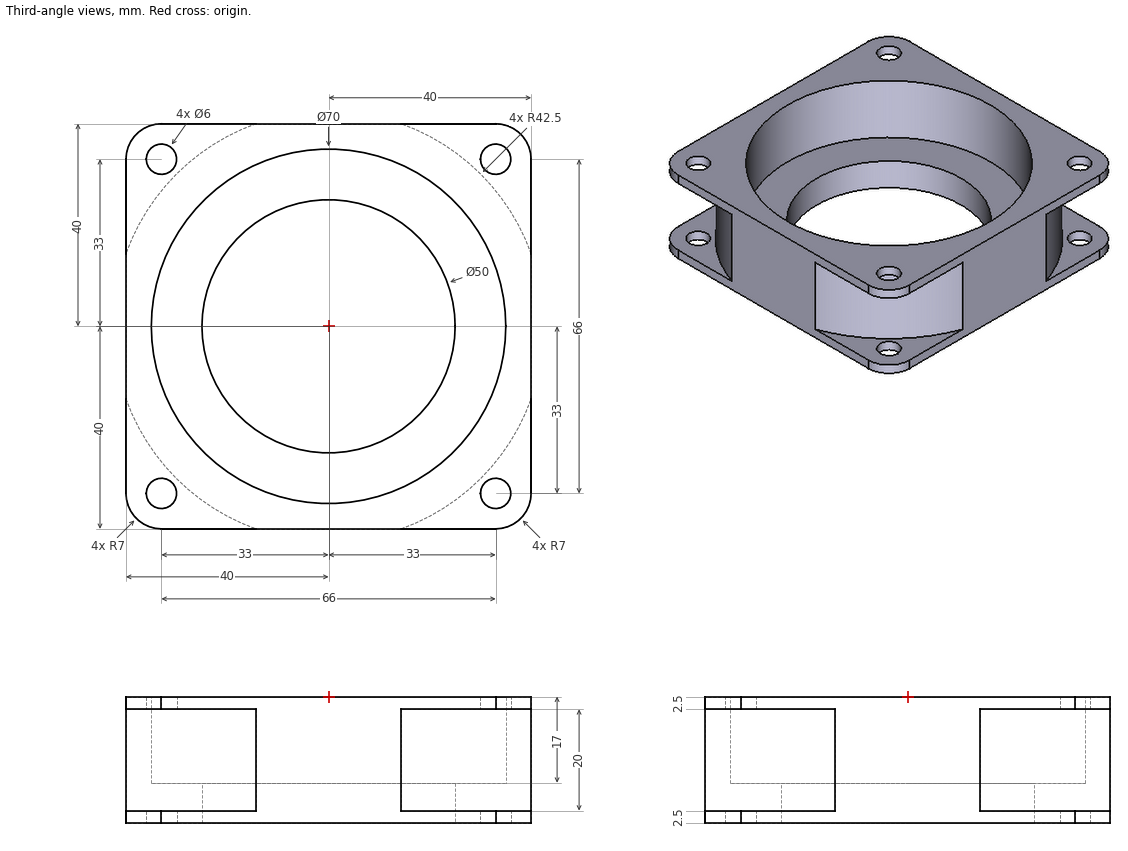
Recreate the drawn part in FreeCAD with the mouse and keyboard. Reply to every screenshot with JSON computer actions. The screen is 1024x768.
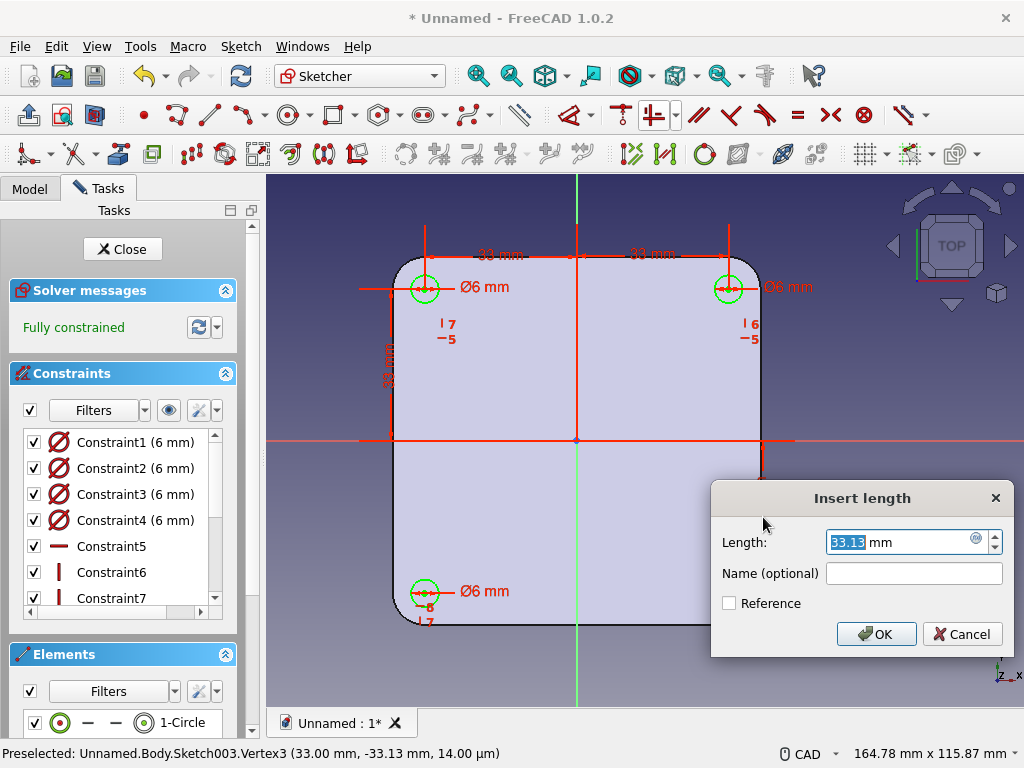
{"action": "type", "text": "33"}
{"action": "key", "text": "Return"}
{"action": "key", "text": "Escape"}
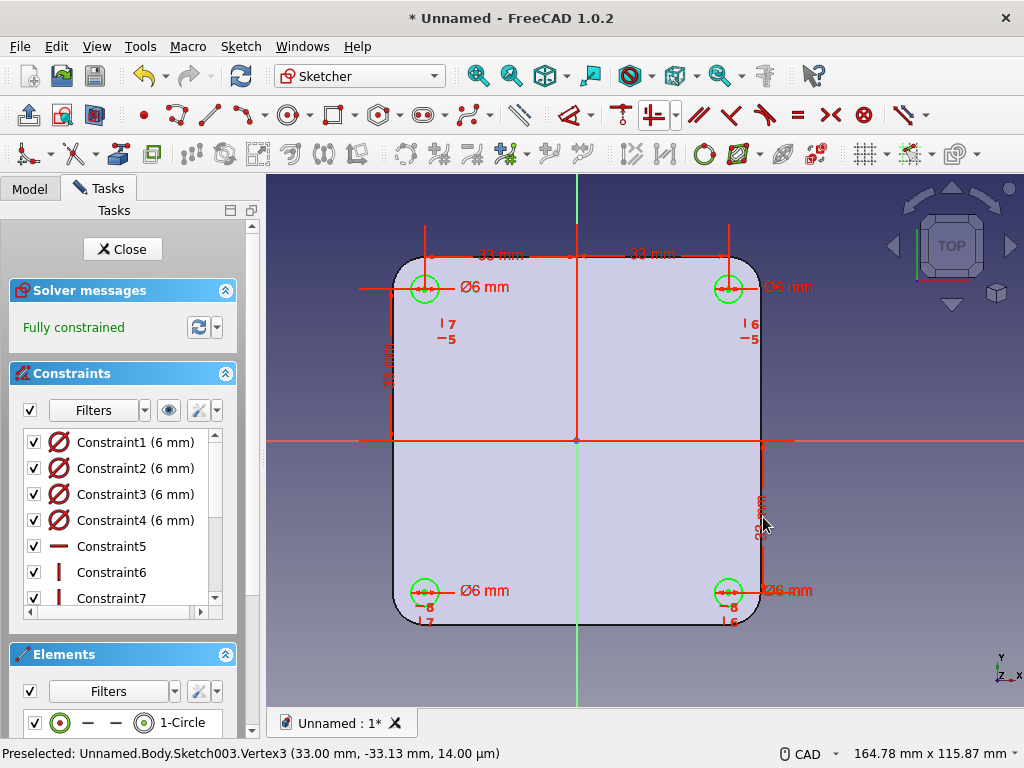
{"action": "left_click", "coordinate": [123, 249]}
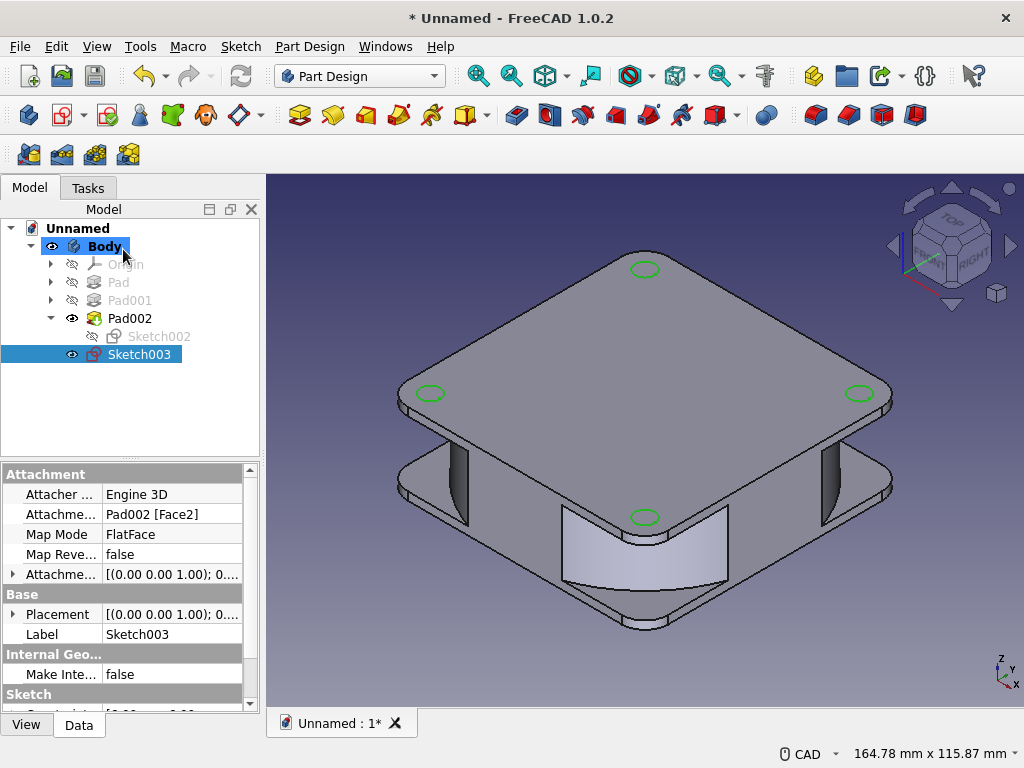
{"action": "left_click", "coordinate": [517, 116]}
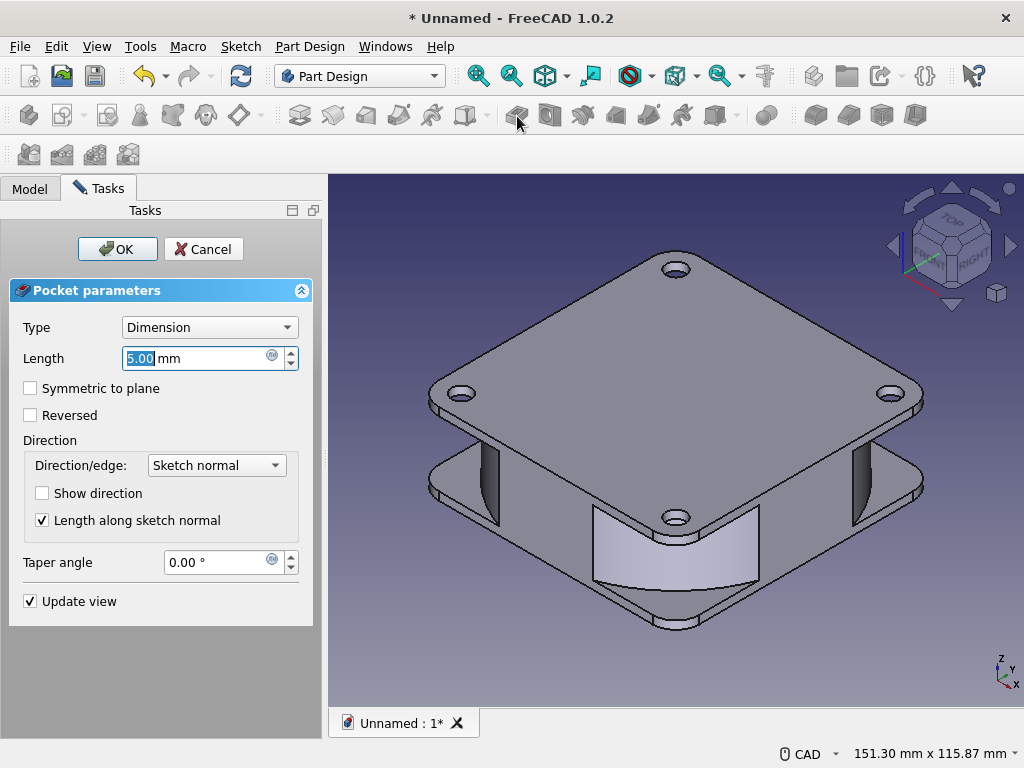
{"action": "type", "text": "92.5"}
{"action": "key", "text": "Tab"}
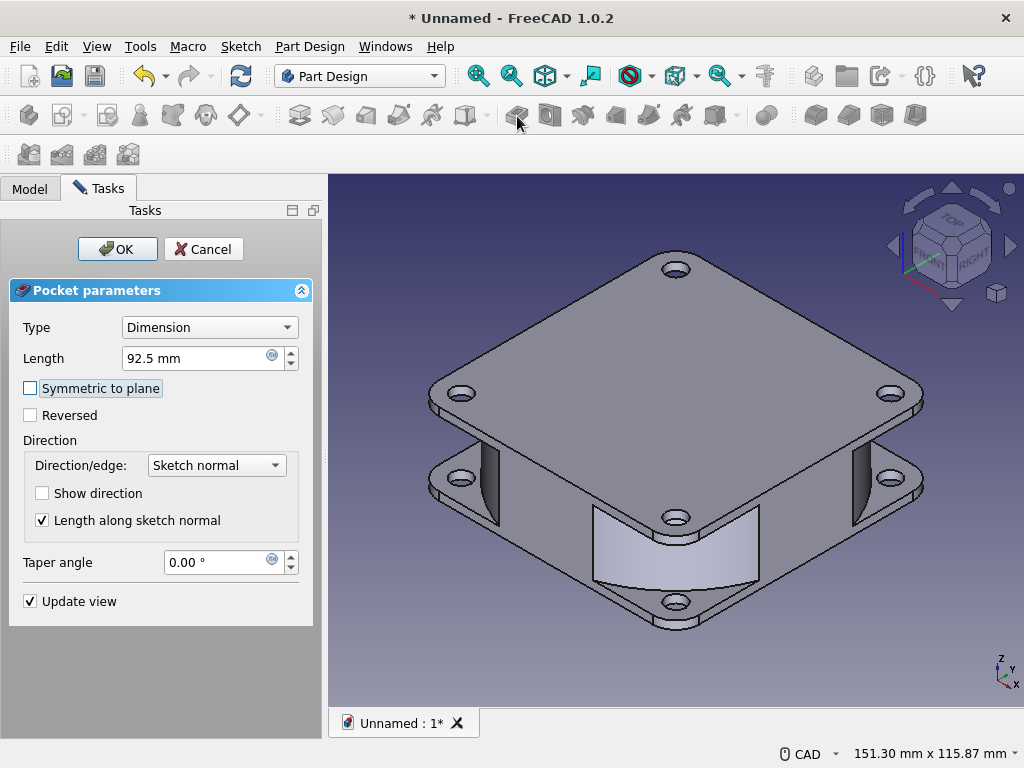
{"action": "left_click", "coordinate": [118, 249]}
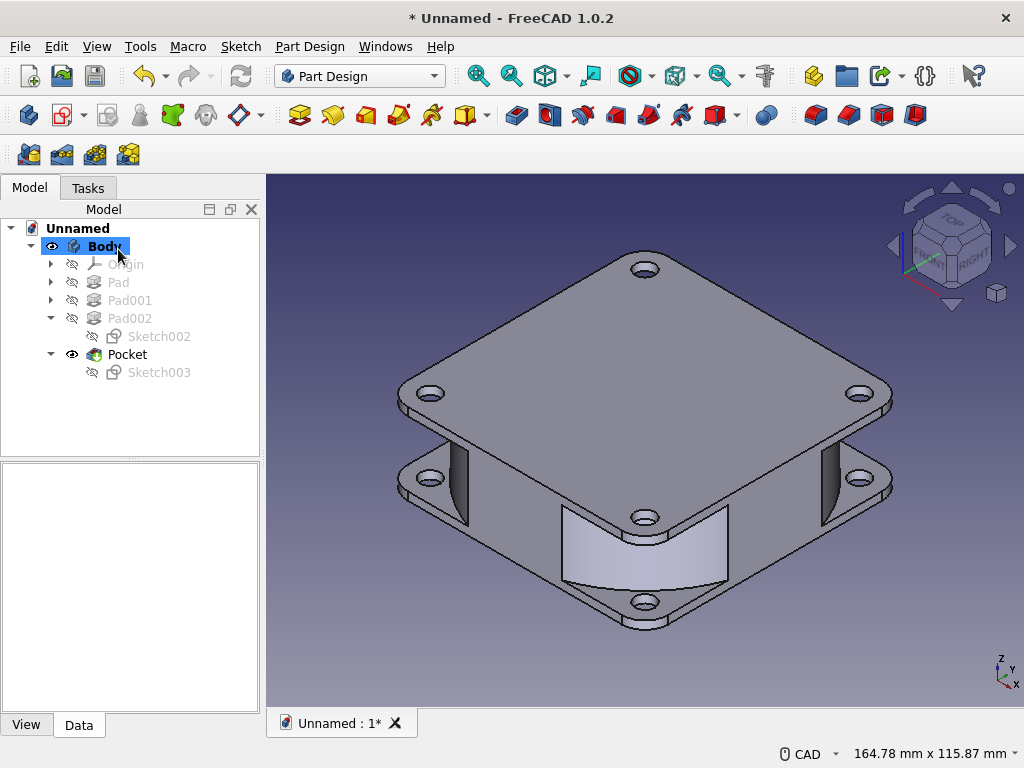
{"action": "left_click", "coordinate": [645, 393]}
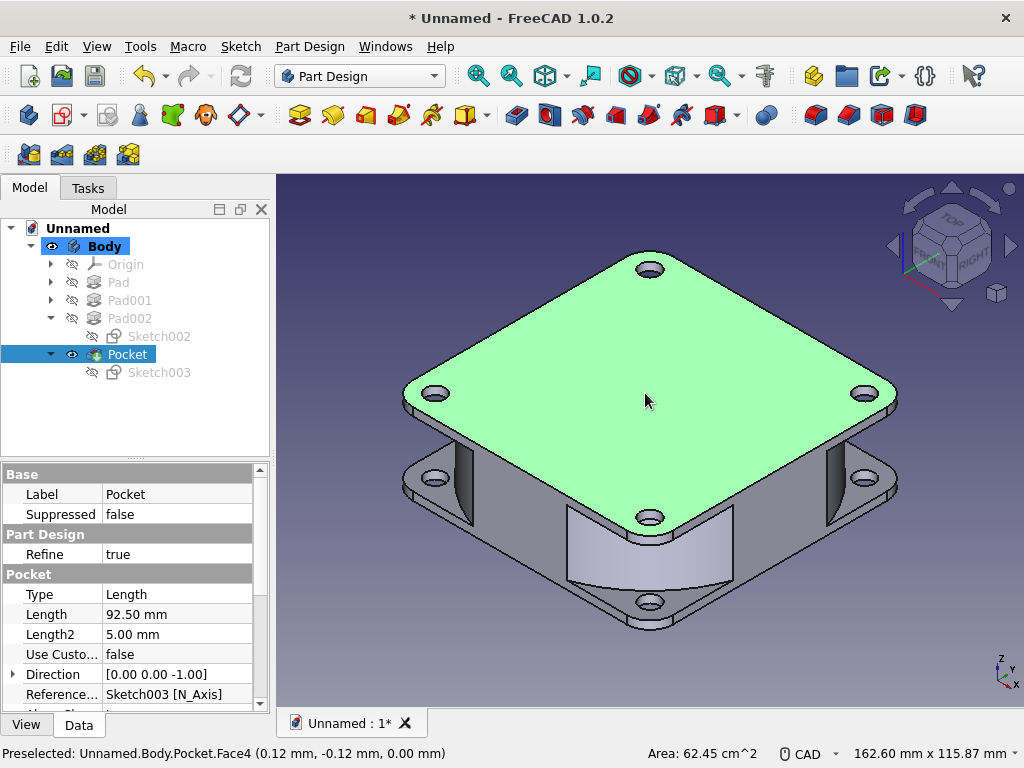
{"action": "left_click", "coordinate": [62, 116]}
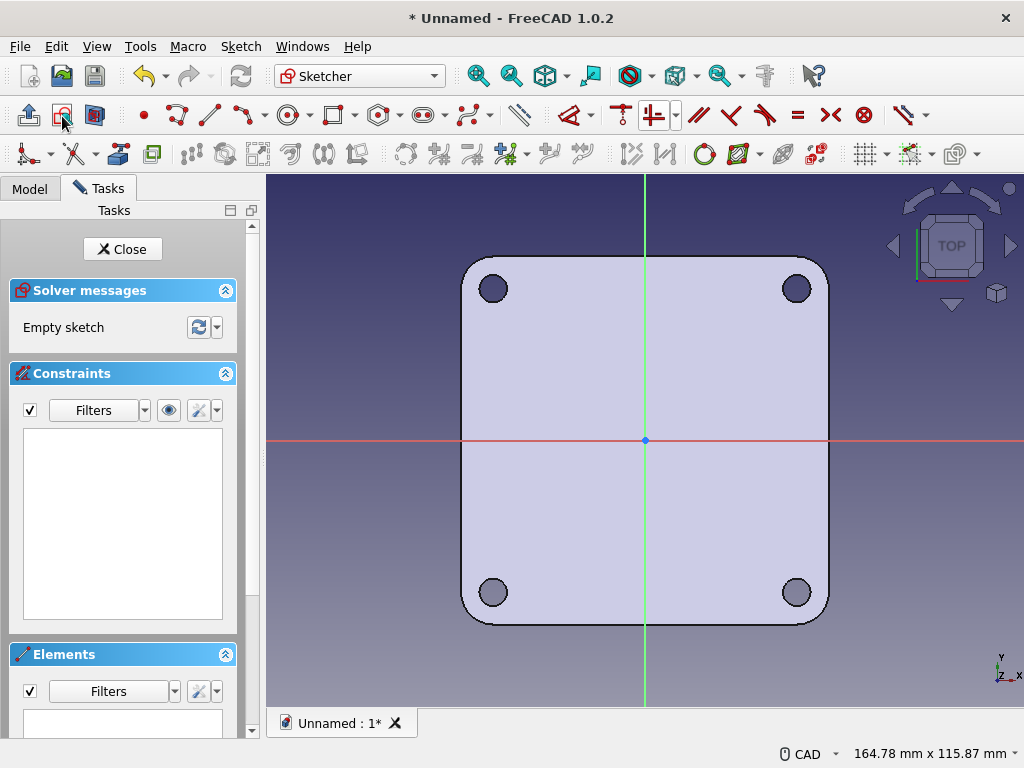
{"action": "scroll", "coordinate": [784, 440], "scroll_direction": "up", "scroll_amount": 2}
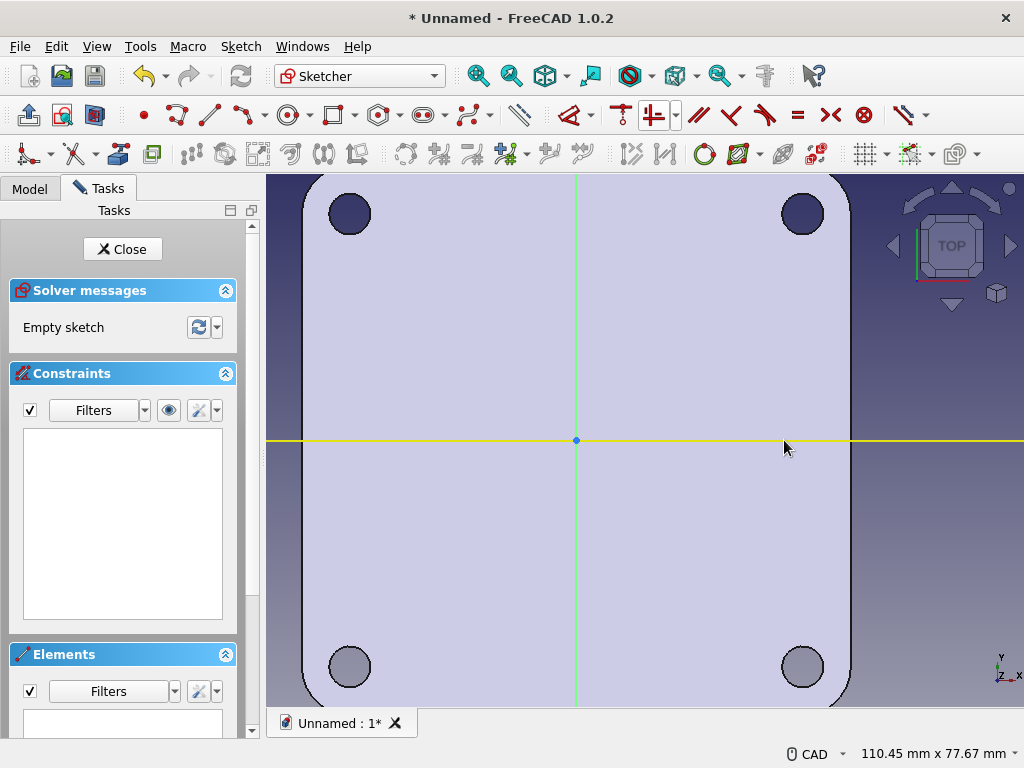
{"action": "left_click", "coordinate": [288, 116]}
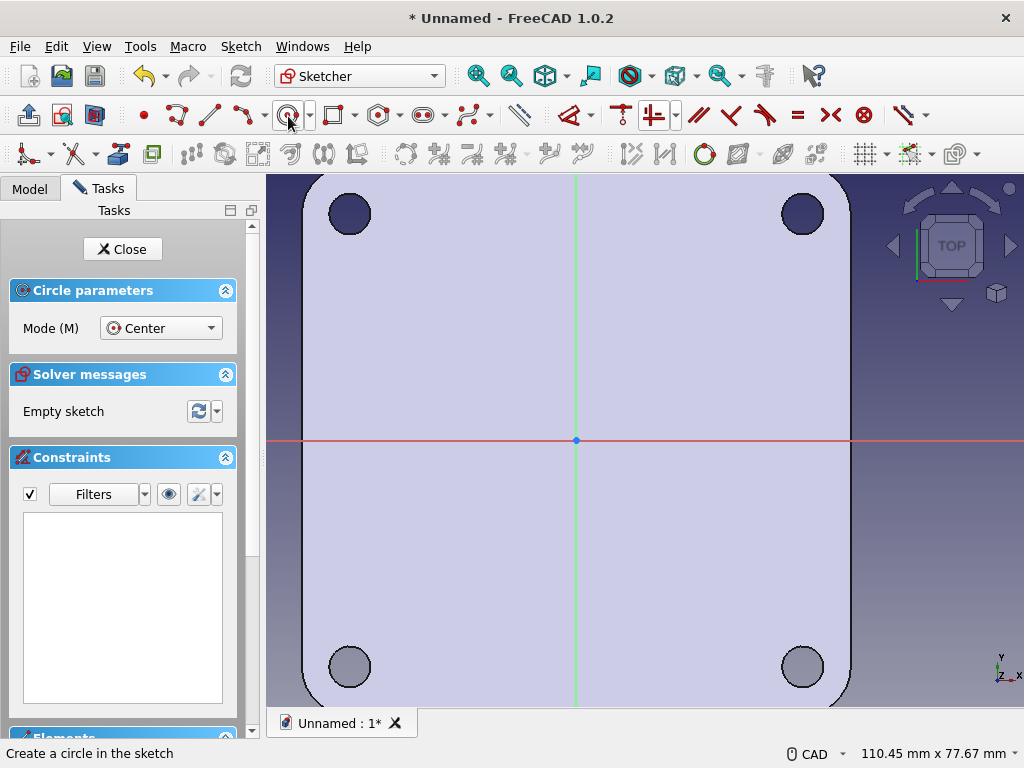
{"action": "left_click", "coordinate": [576, 440]}
{"action": "mouse_move", "coordinate": [698, 319]}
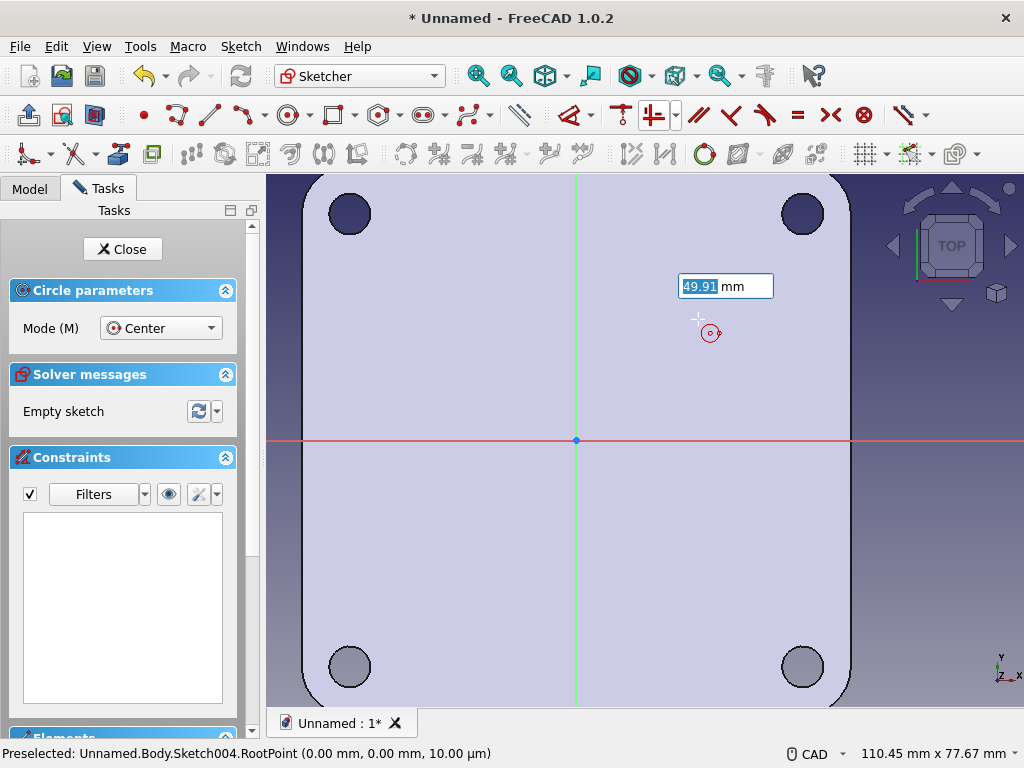
{"action": "type", "text": "50"}
{"action": "key", "text": "Return"}
{"action": "key", "text": "Escape"}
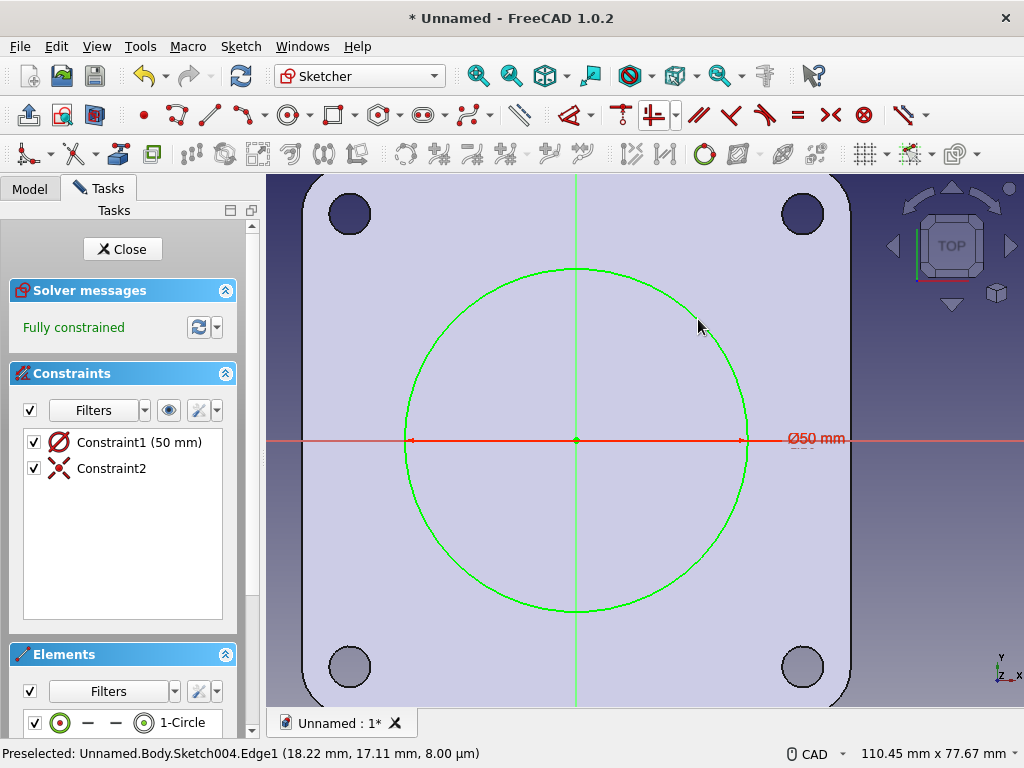
{"action": "left_click", "coordinate": [123, 249]}